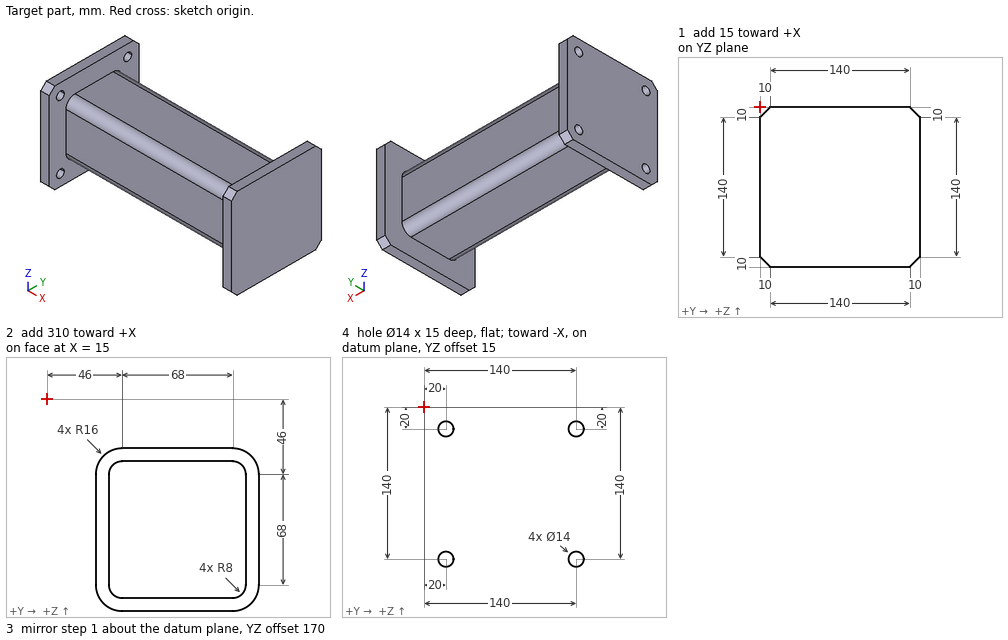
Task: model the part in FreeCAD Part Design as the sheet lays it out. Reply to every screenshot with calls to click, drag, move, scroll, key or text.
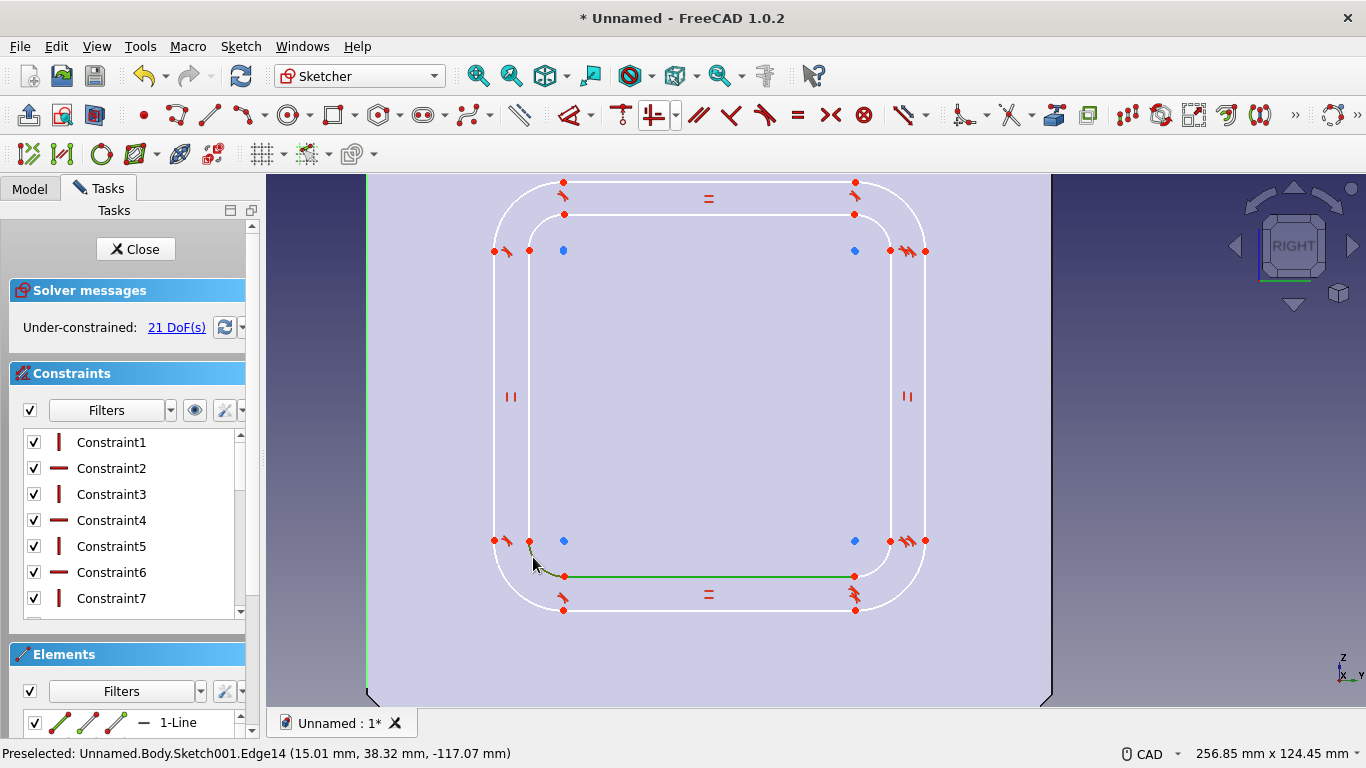
click(765, 116)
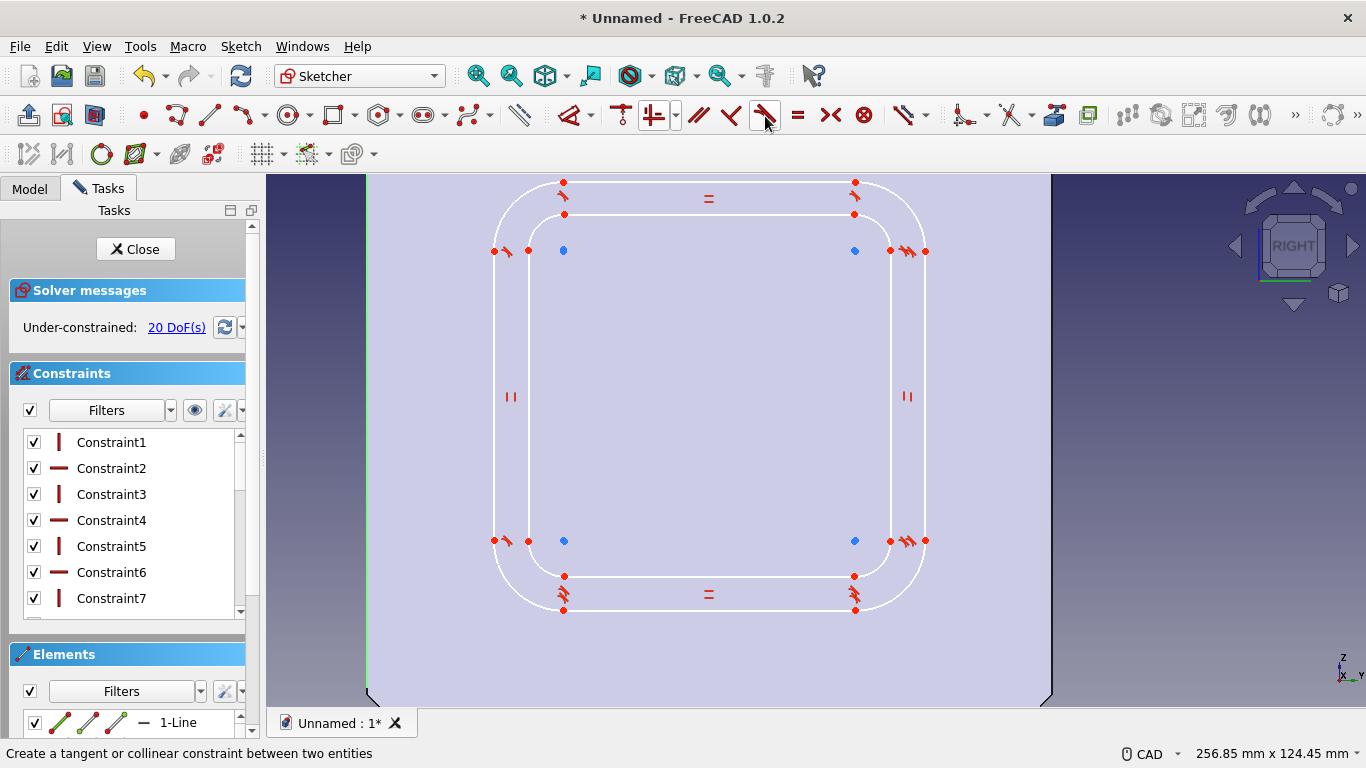
click(529, 454)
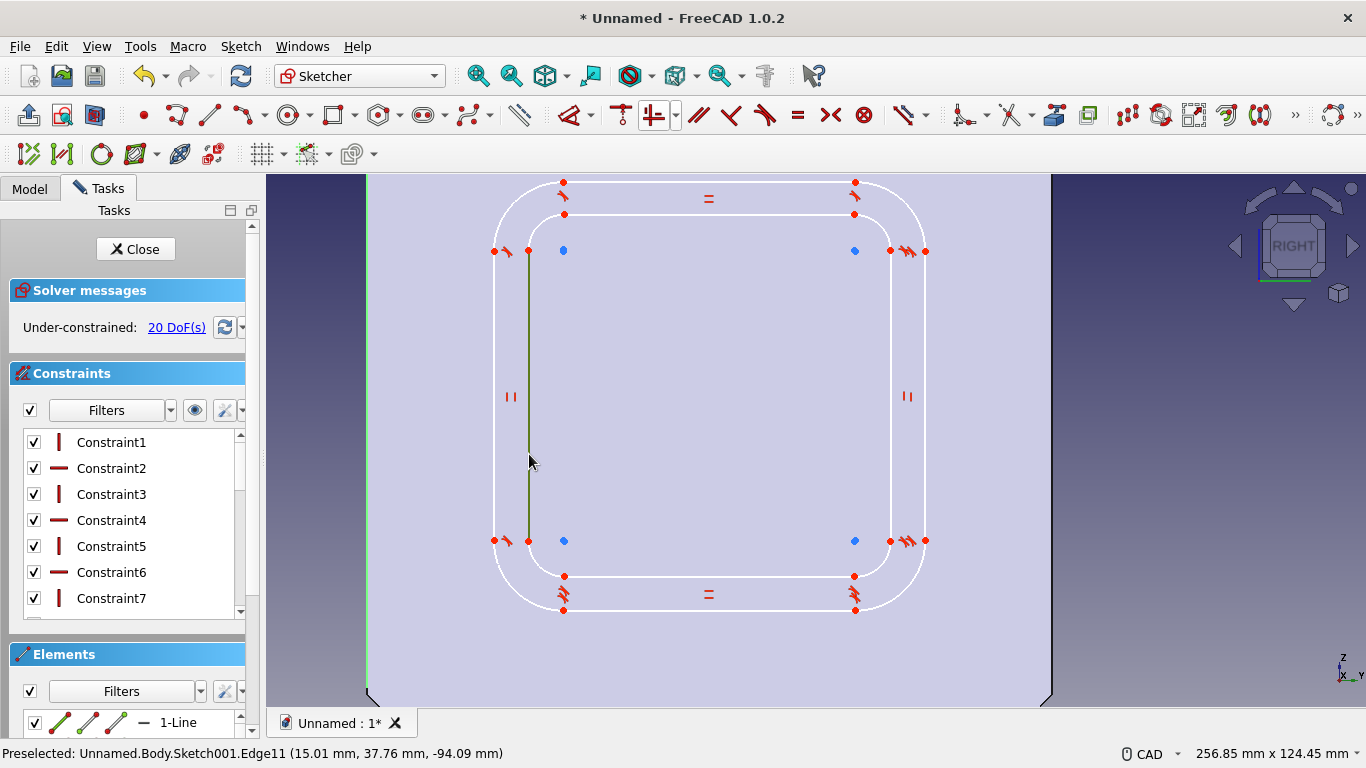
click(533, 558)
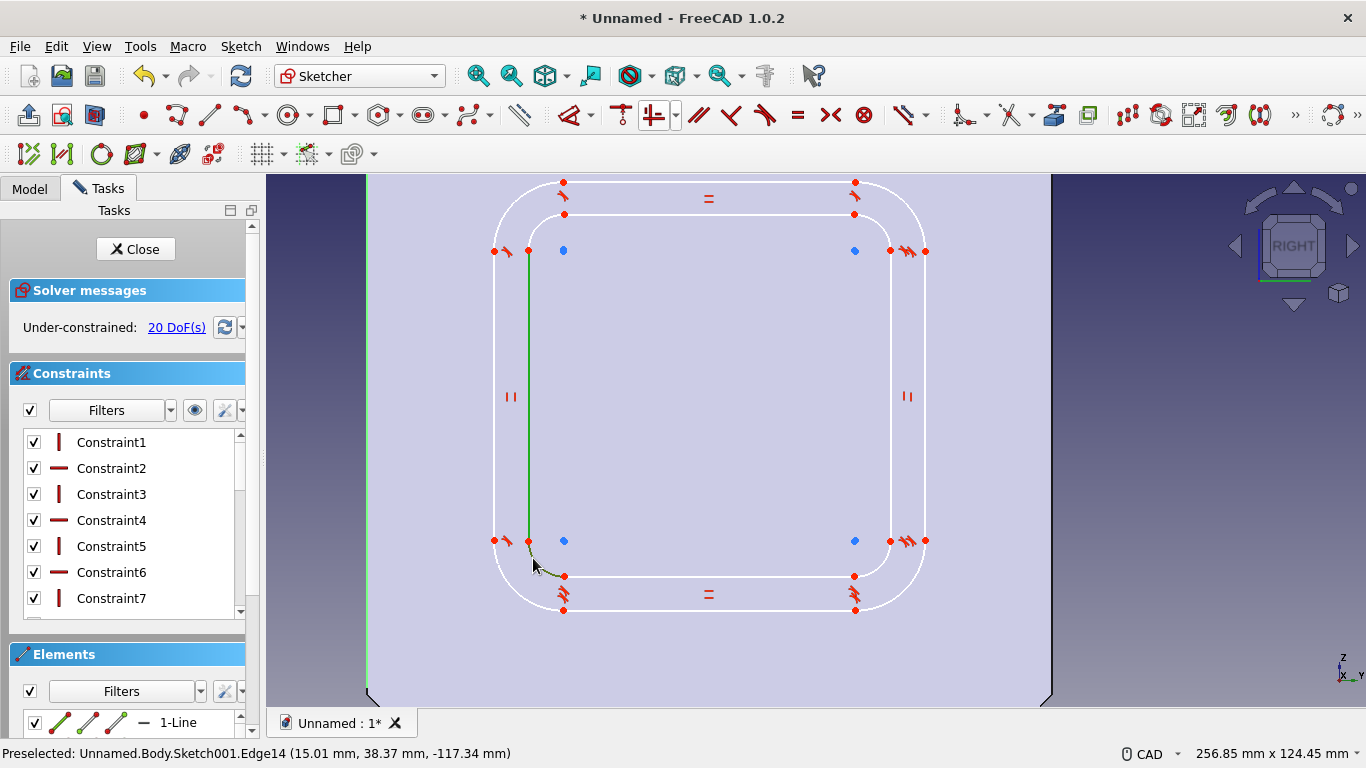
click(765, 116)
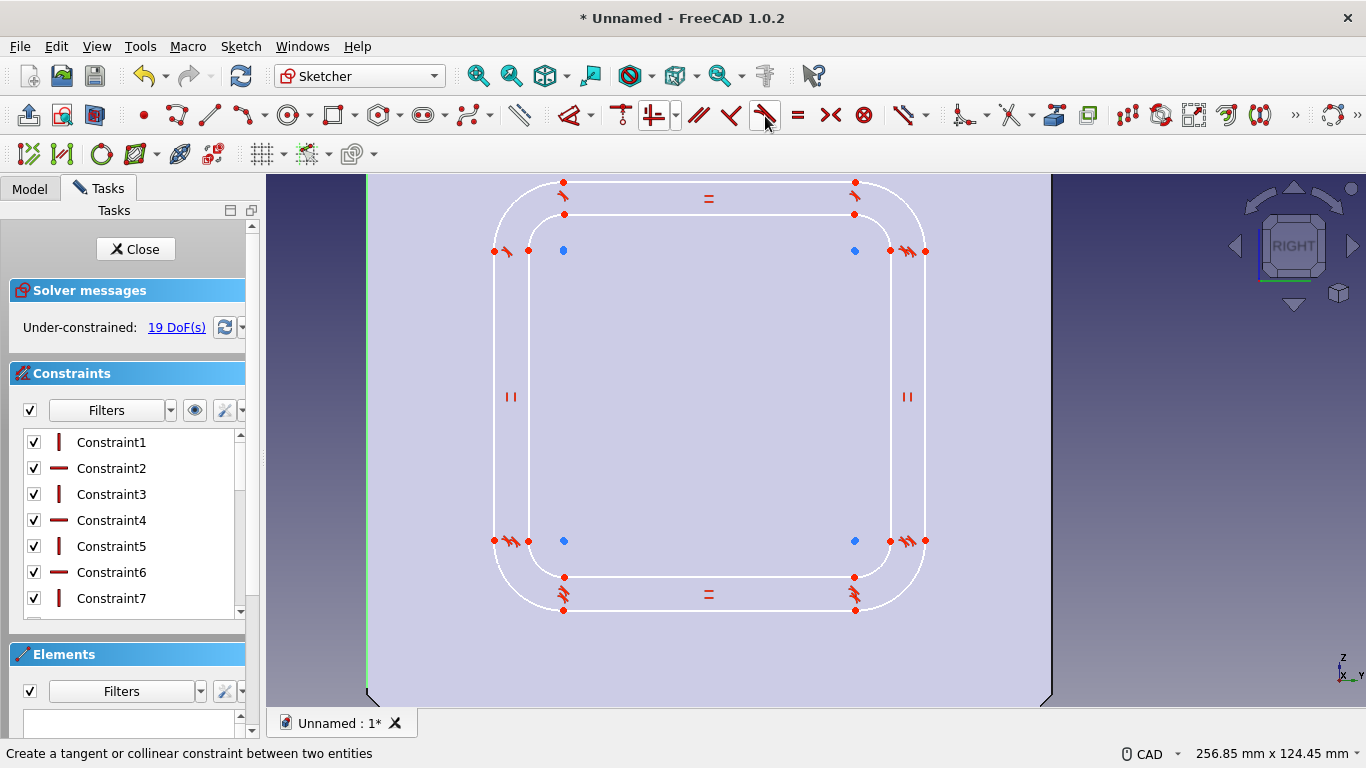
click(529, 454)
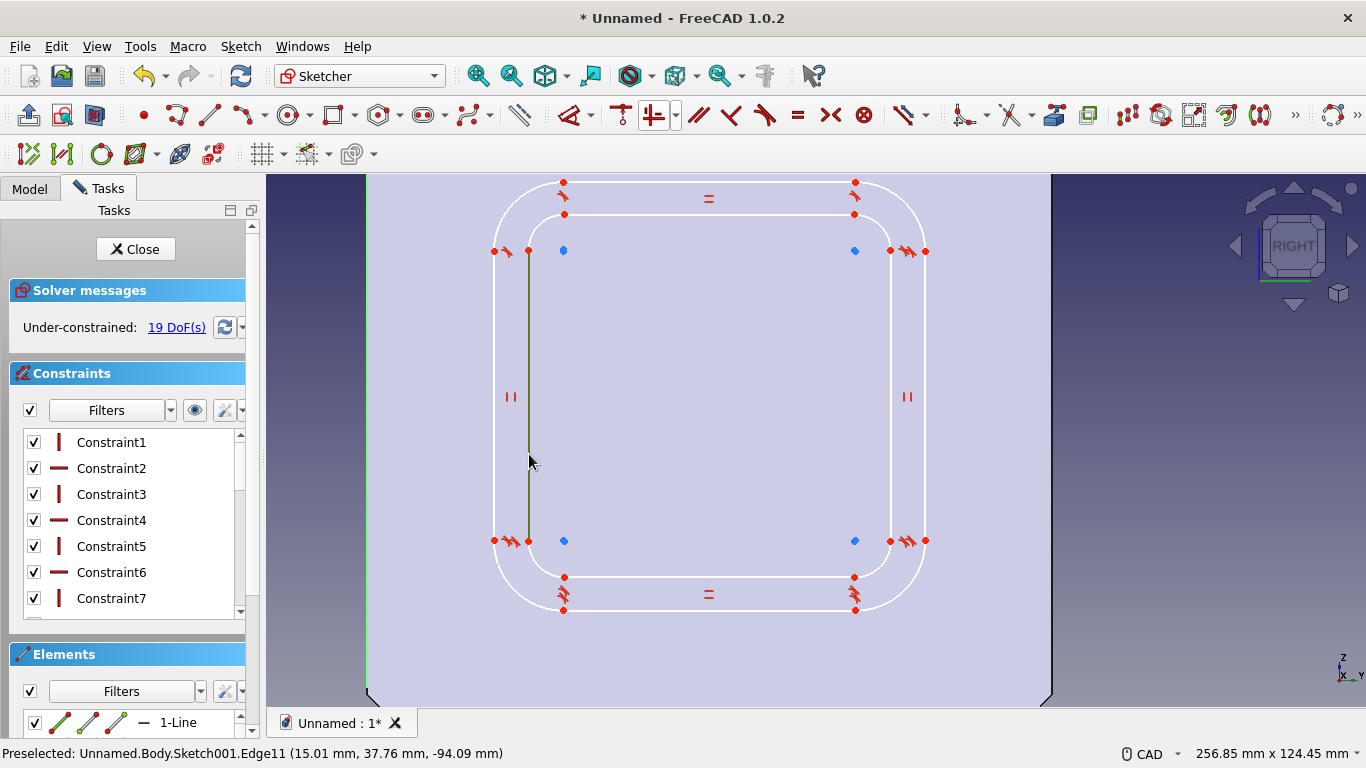
click(548, 219)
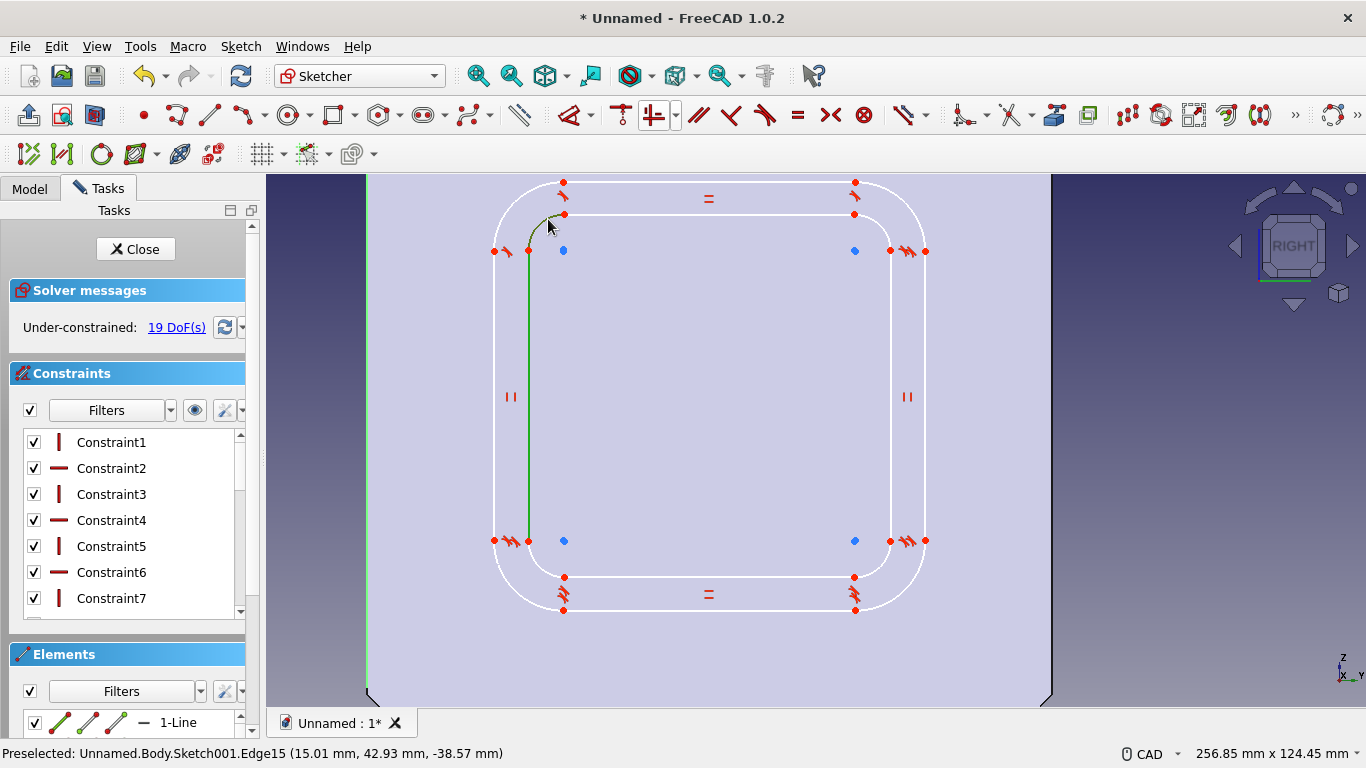
click(765, 116)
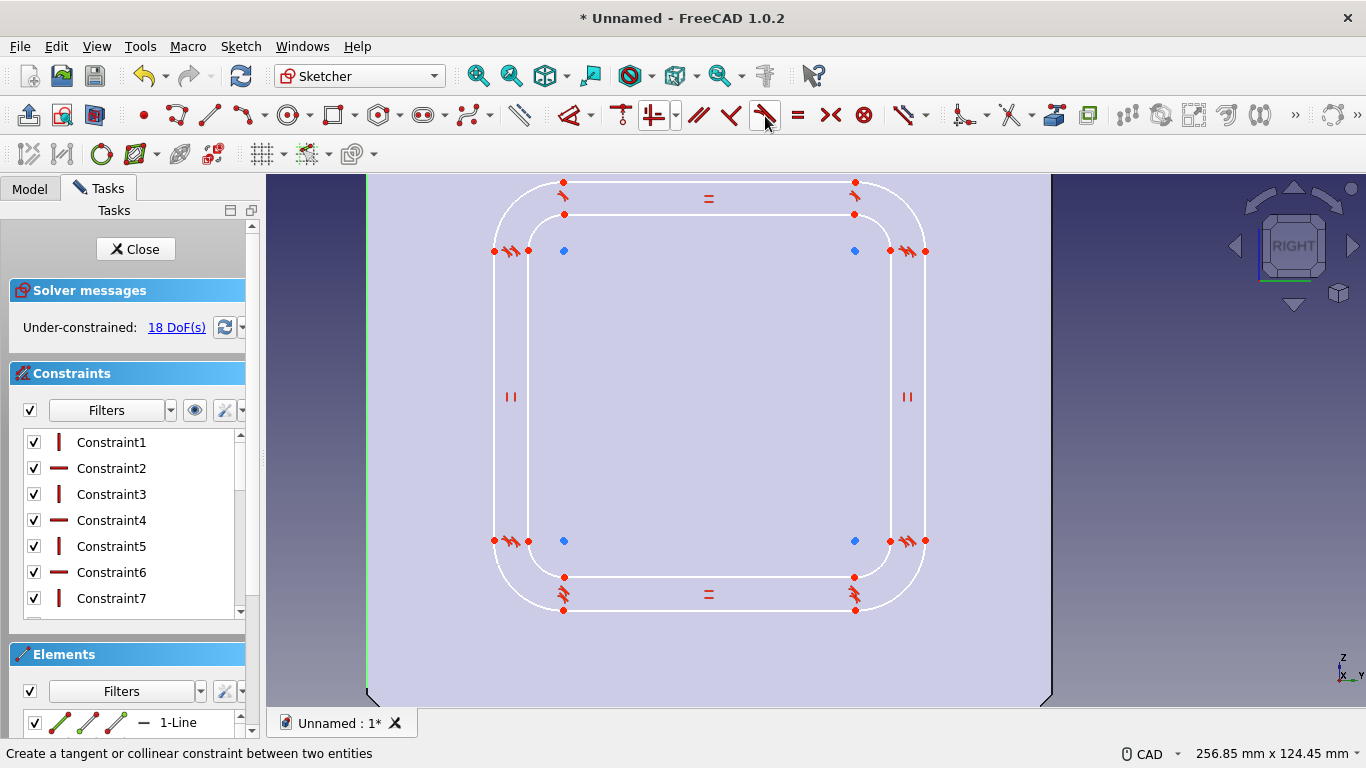
click(651, 215)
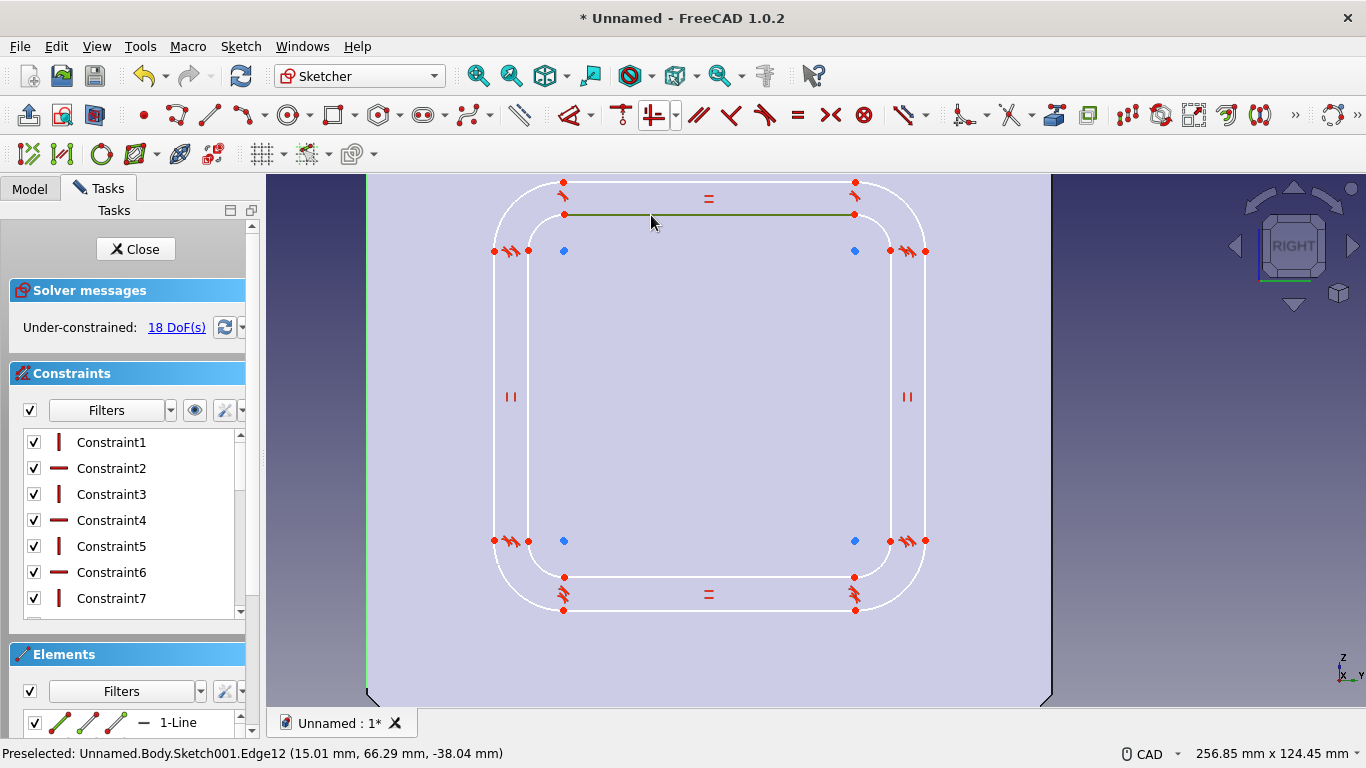
click(548, 219)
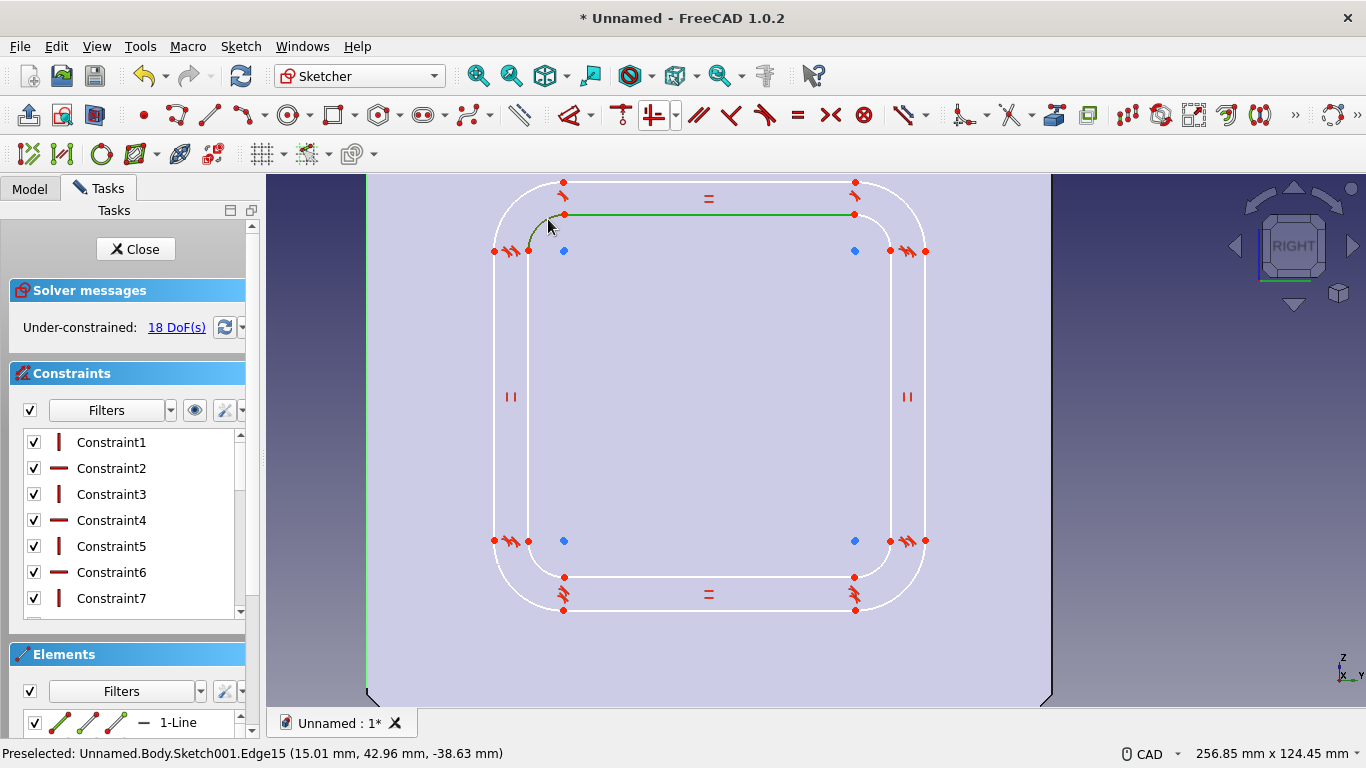
click(765, 116)